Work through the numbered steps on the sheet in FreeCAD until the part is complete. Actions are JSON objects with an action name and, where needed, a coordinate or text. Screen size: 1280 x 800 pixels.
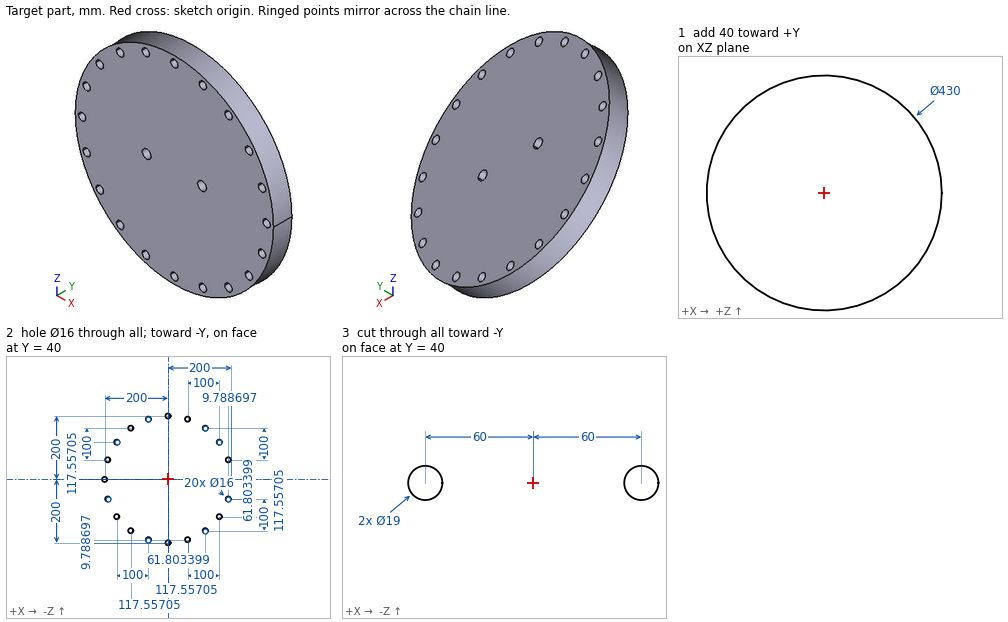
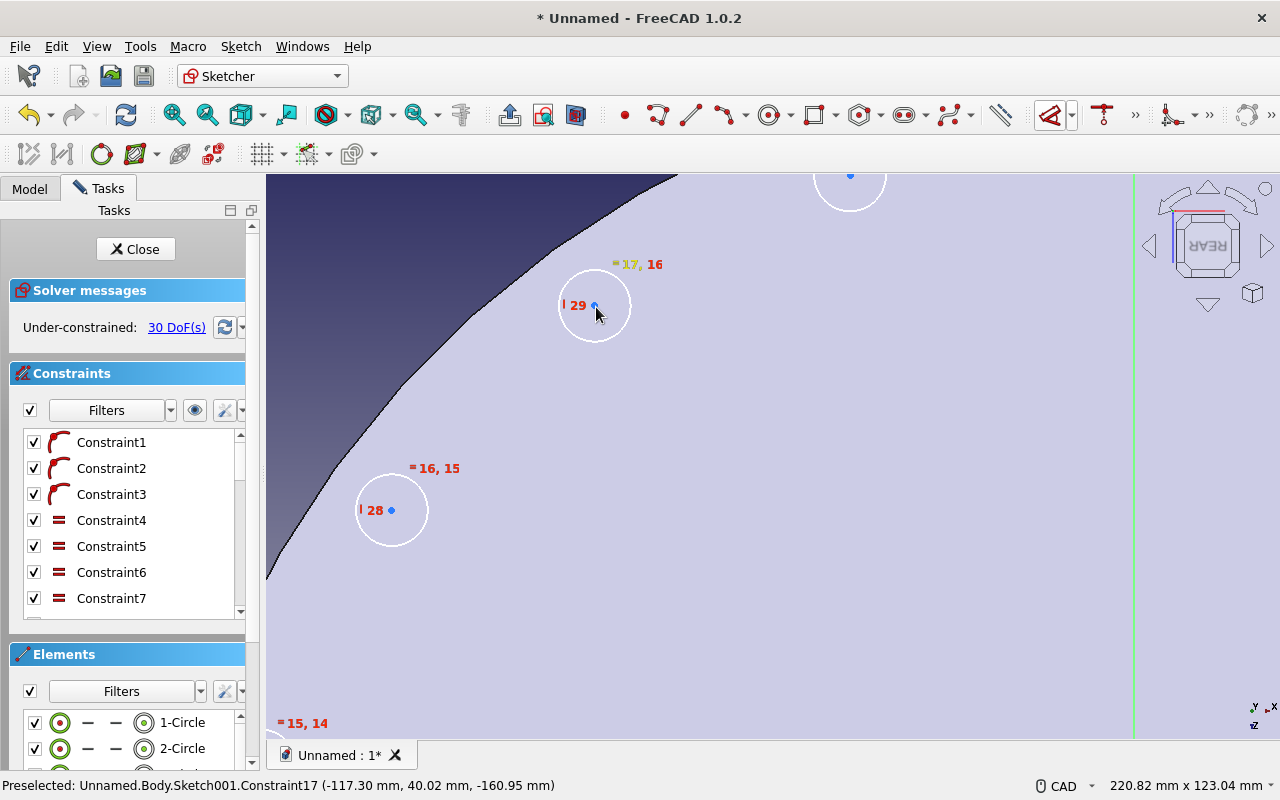
{"action": "left_click", "coordinate": [595, 306]}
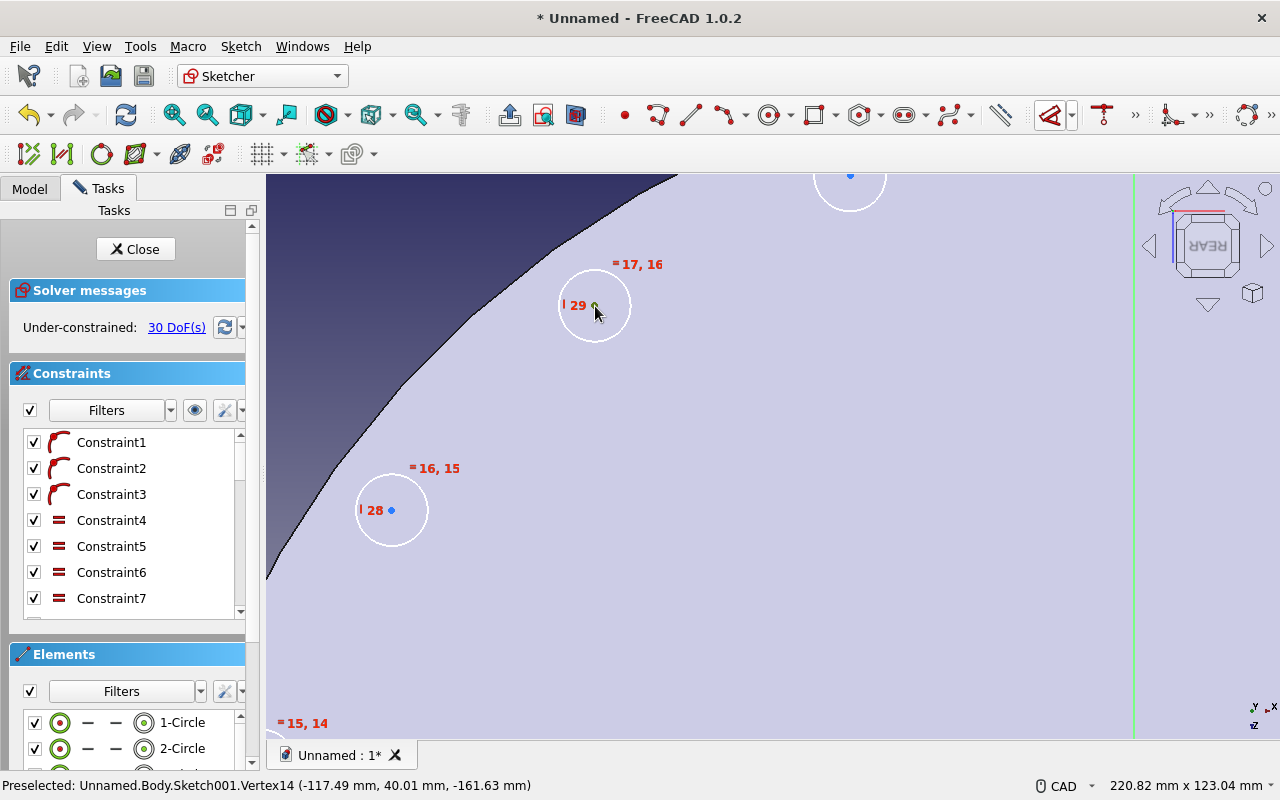
{"action": "scroll", "coordinate": [596, 307], "scroll_direction": "down", "scroll_amount": 8}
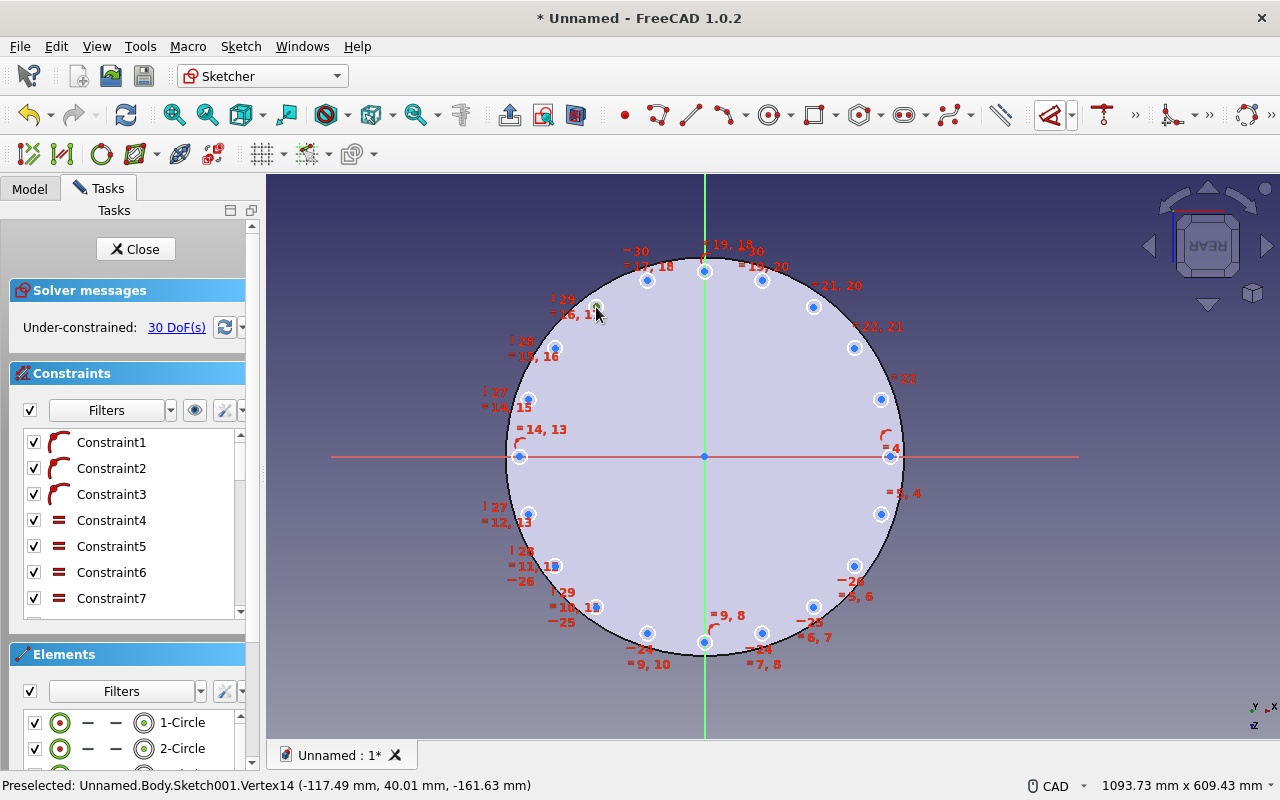
{"action": "left_click", "coordinate": [814, 307]}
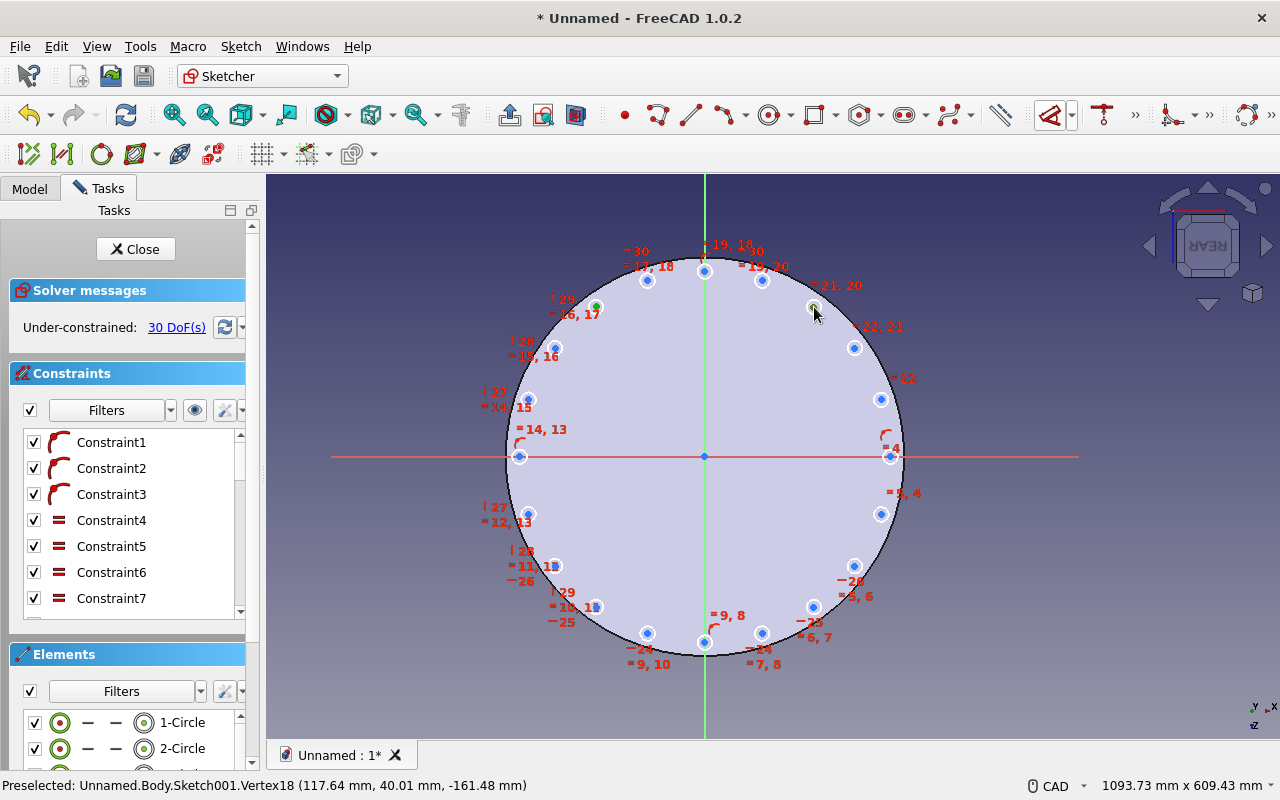
{"action": "key", "text": "h"}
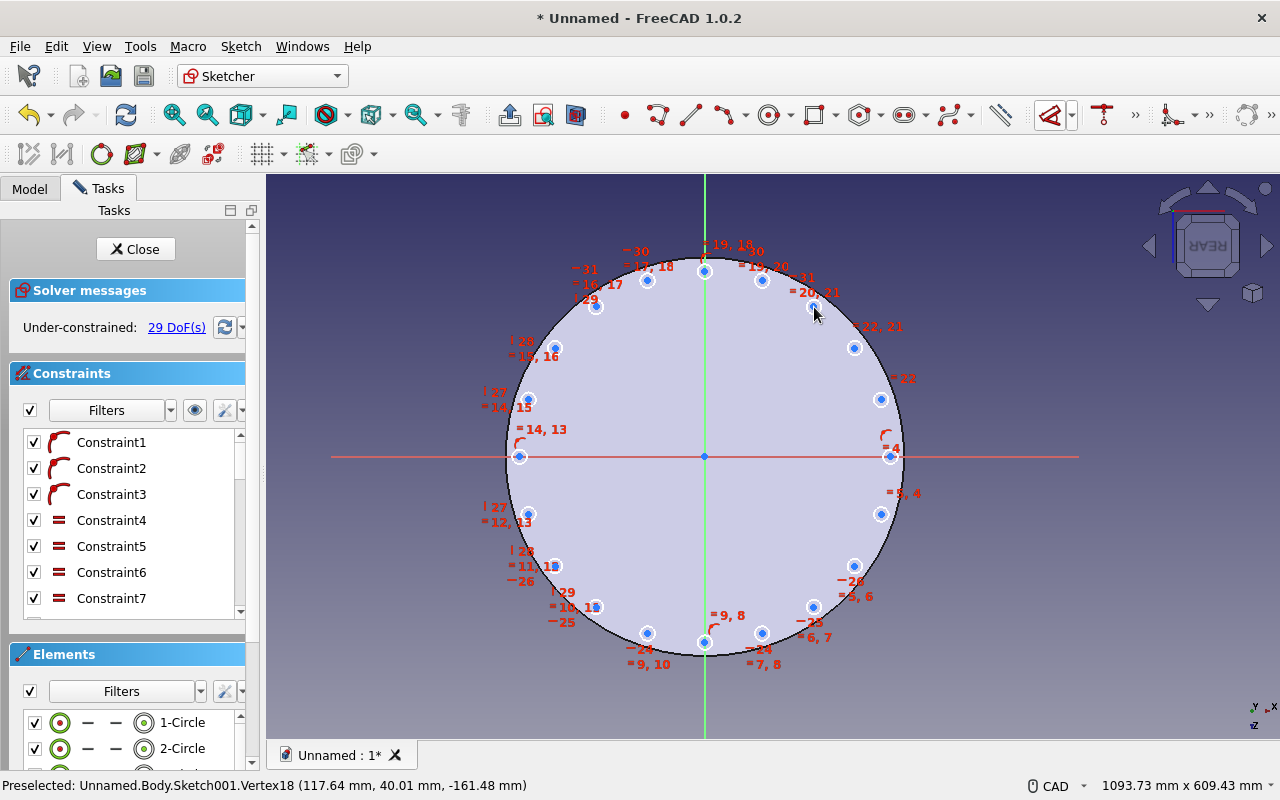
{"action": "left_click", "coordinate": [855, 566]}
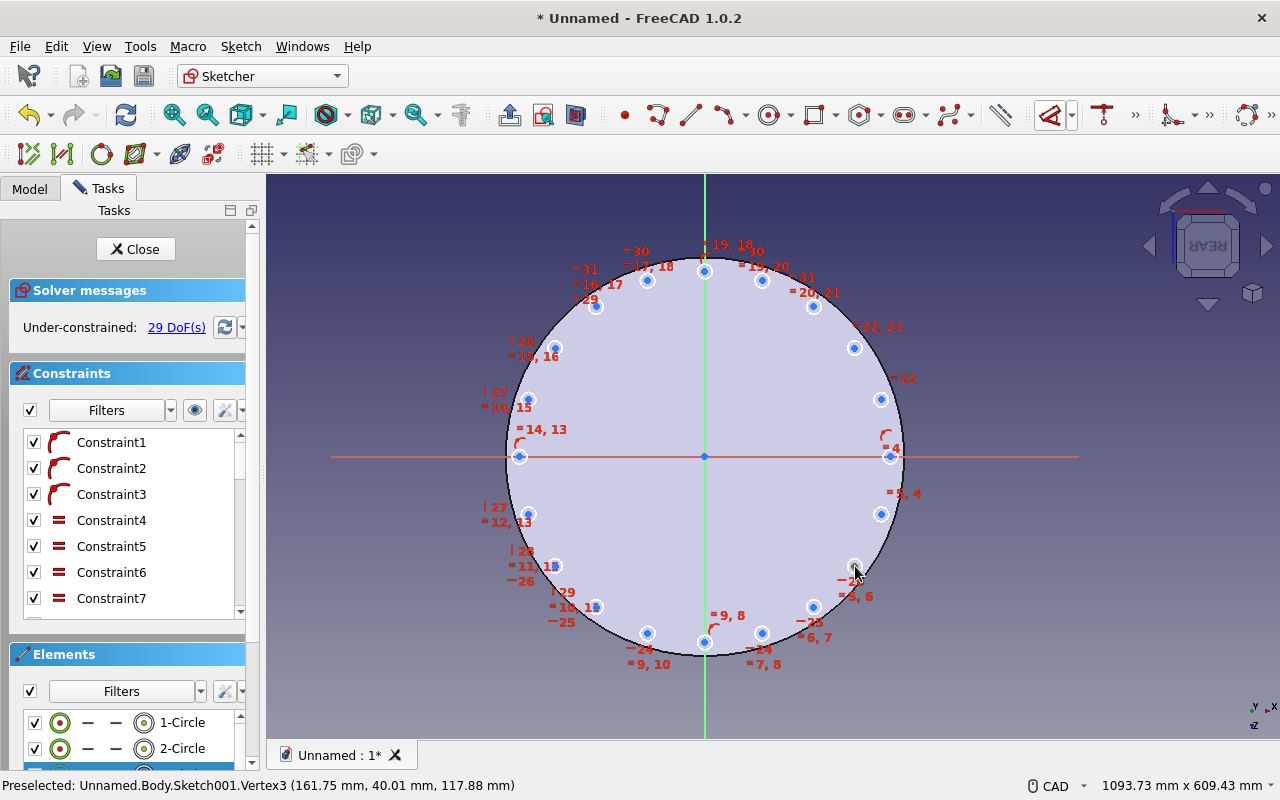
{"action": "left_click", "coordinate": [855, 348]}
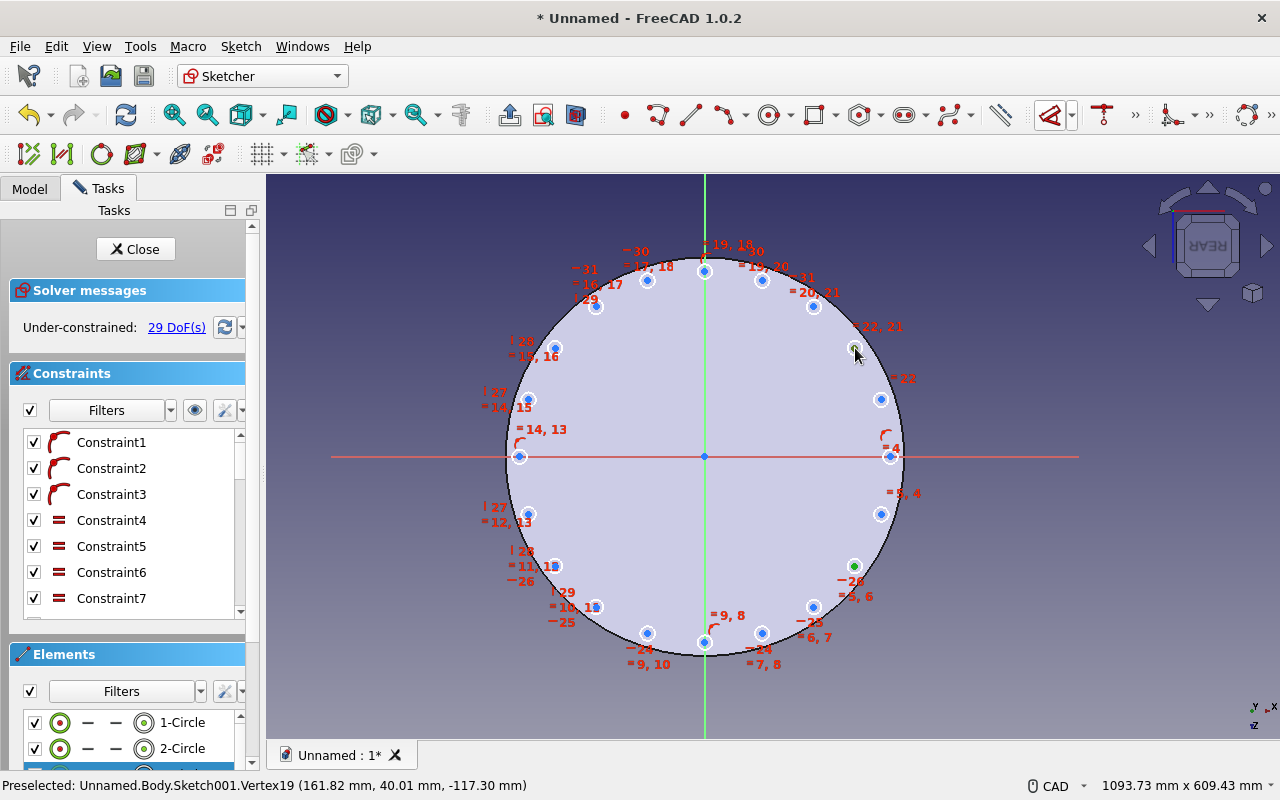
{"action": "key", "text": "v"}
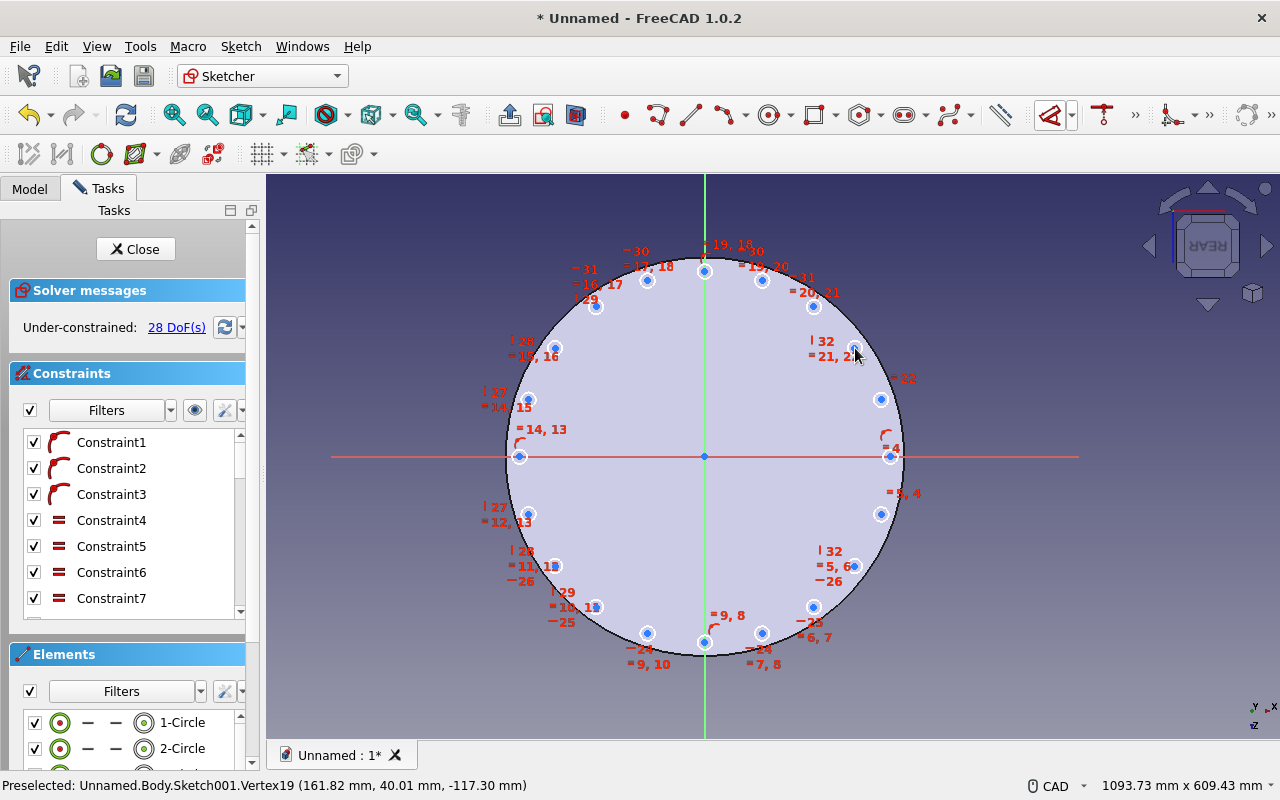
{"action": "left_click", "coordinate": [881, 514]}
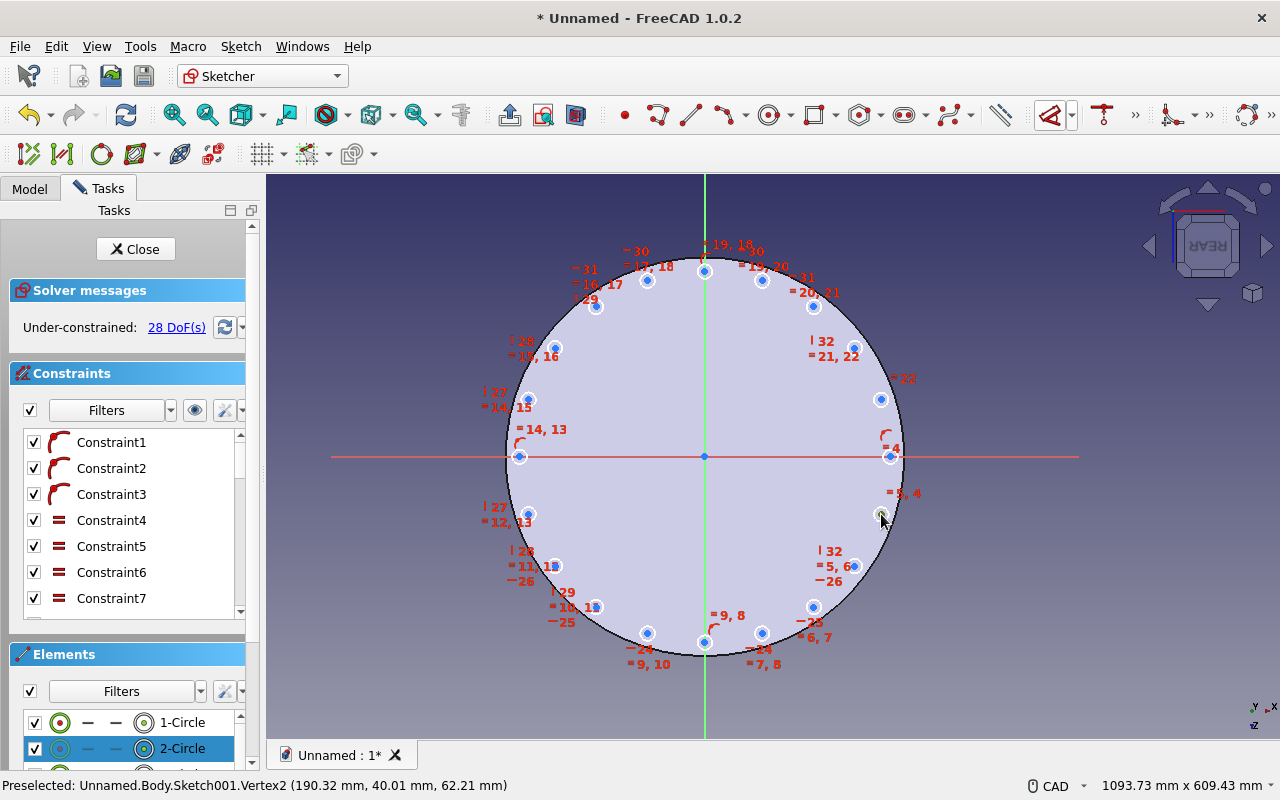
{"action": "left_click", "coordinate": [881, 400]}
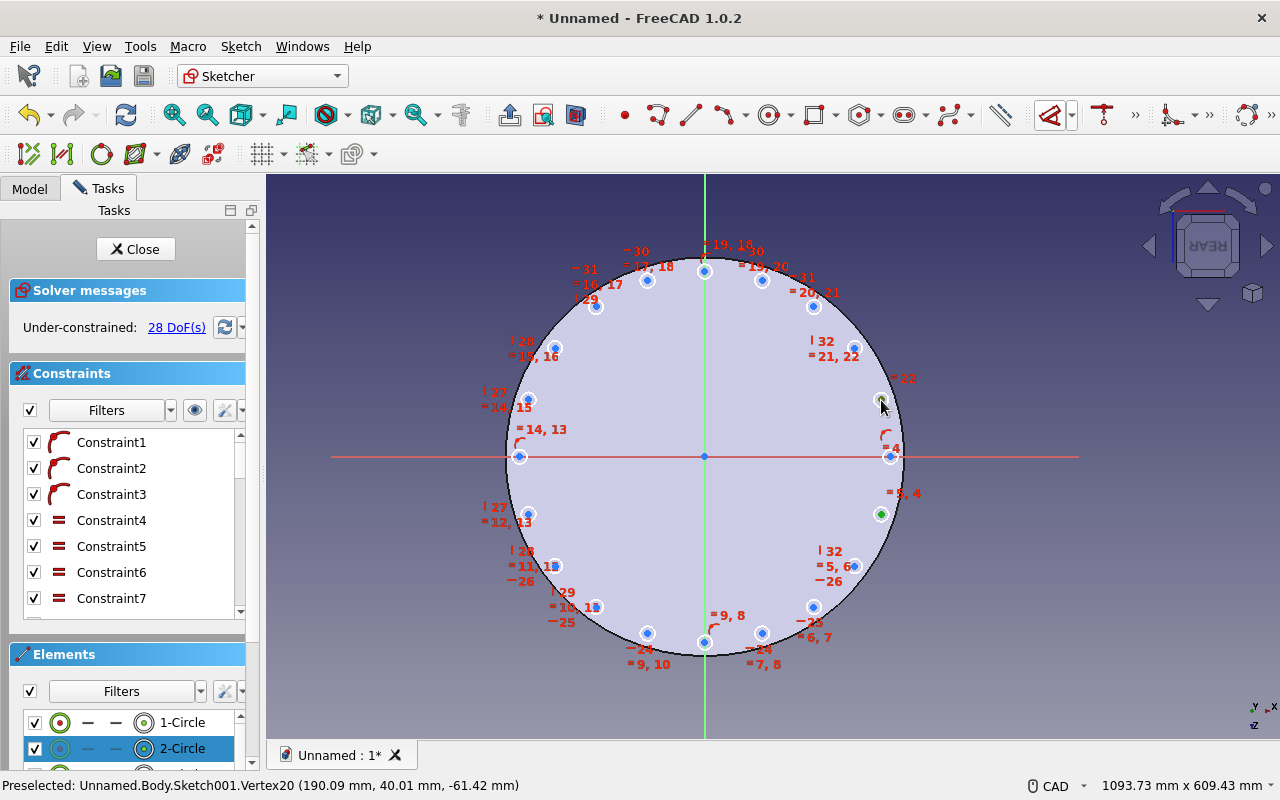
{"action": "key", "text": "v"}